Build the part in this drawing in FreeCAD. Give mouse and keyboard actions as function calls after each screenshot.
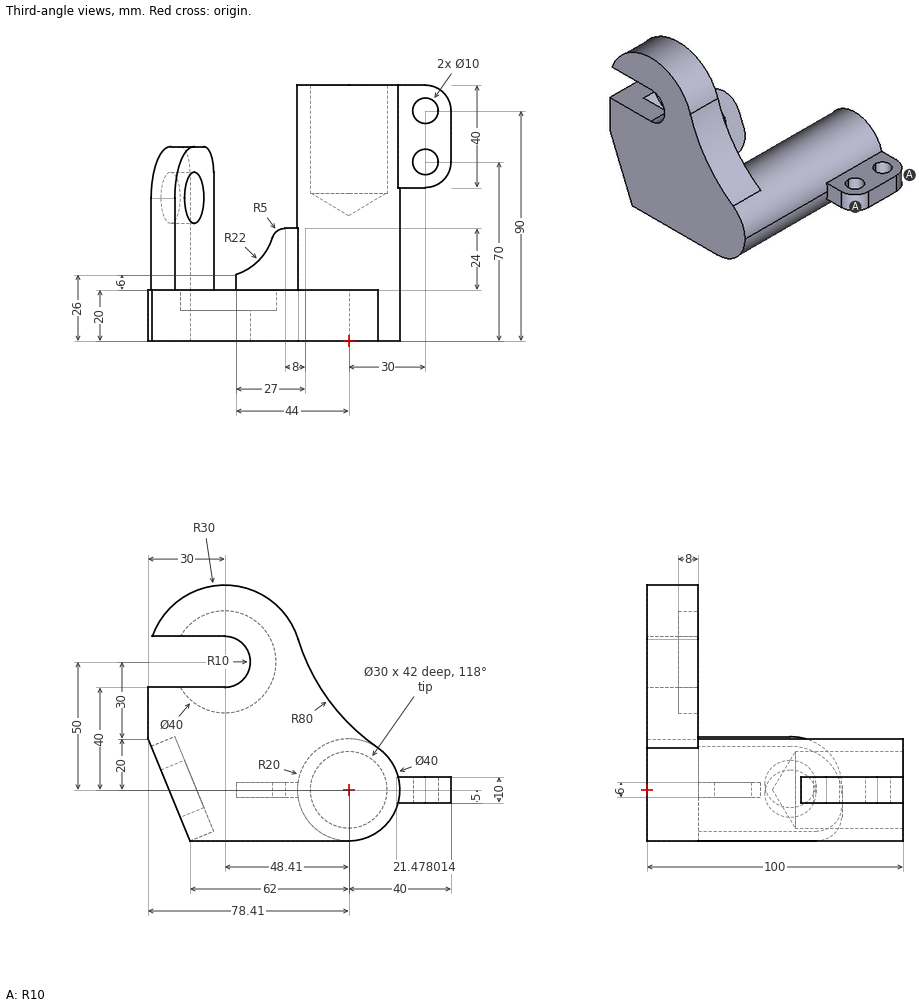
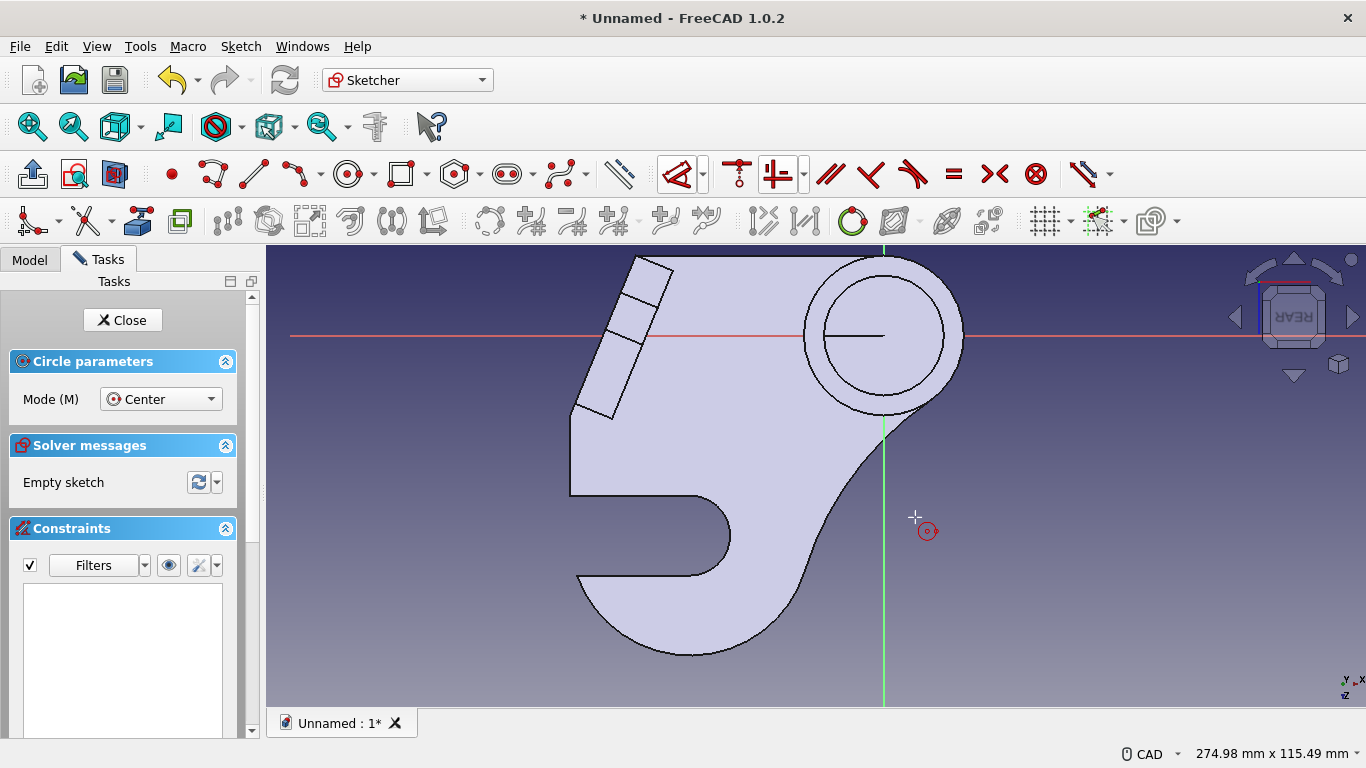
click(690, 536)
click(747, 479)
key(Escape)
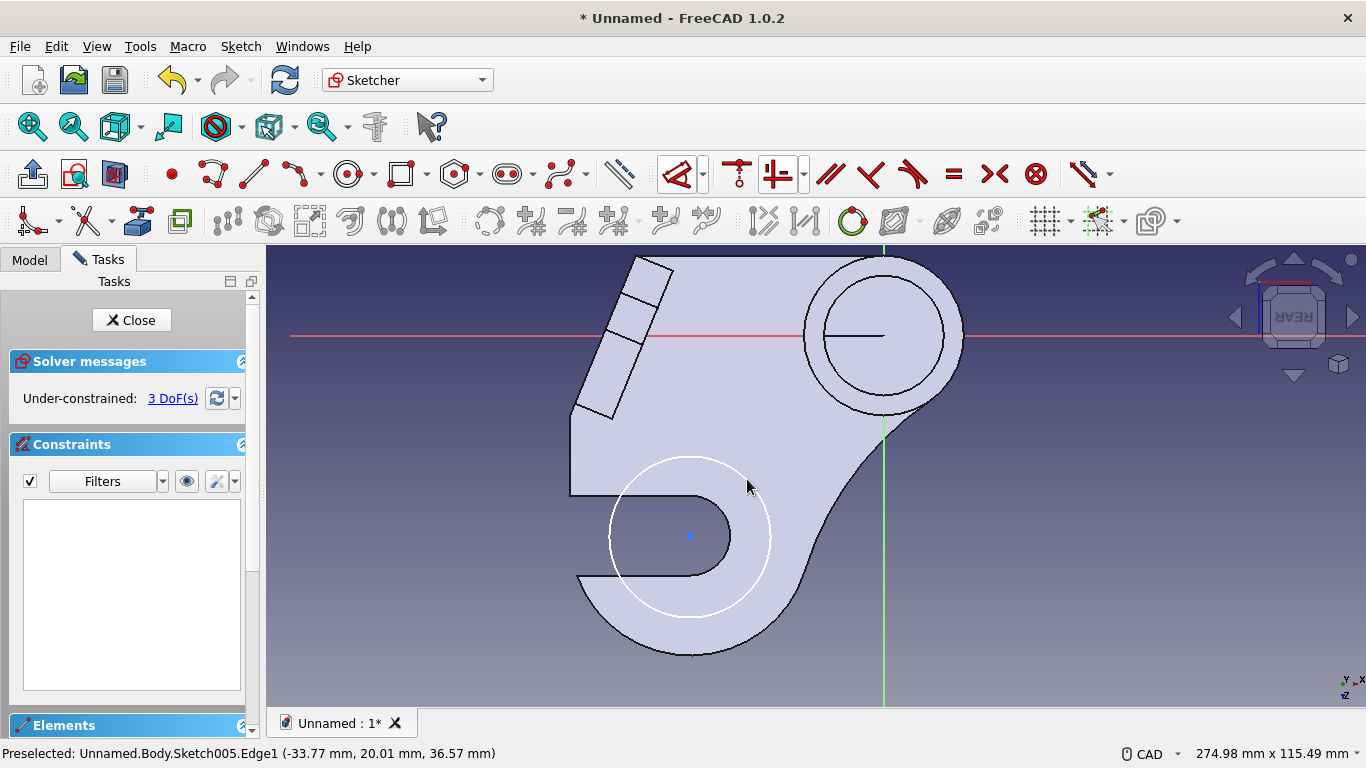
key(d)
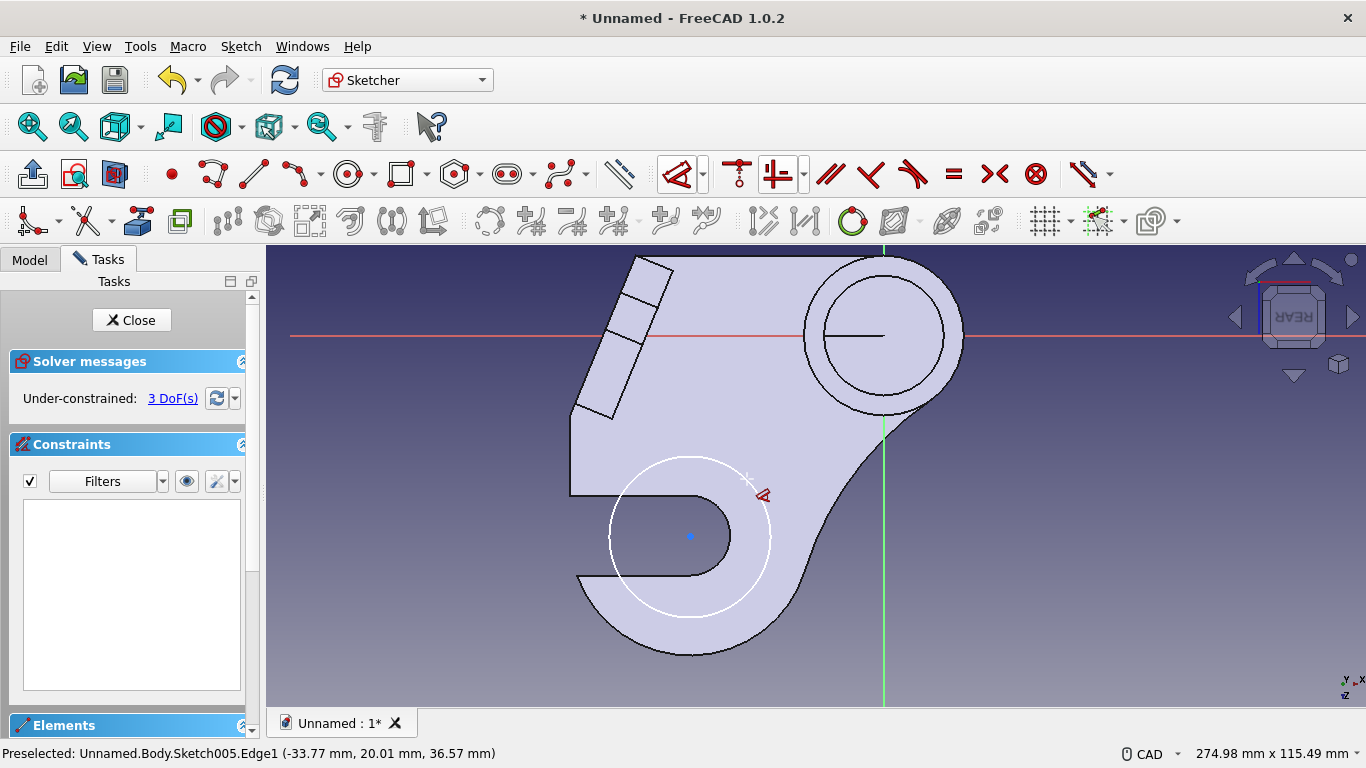
click(747, 480)
click(770, 457)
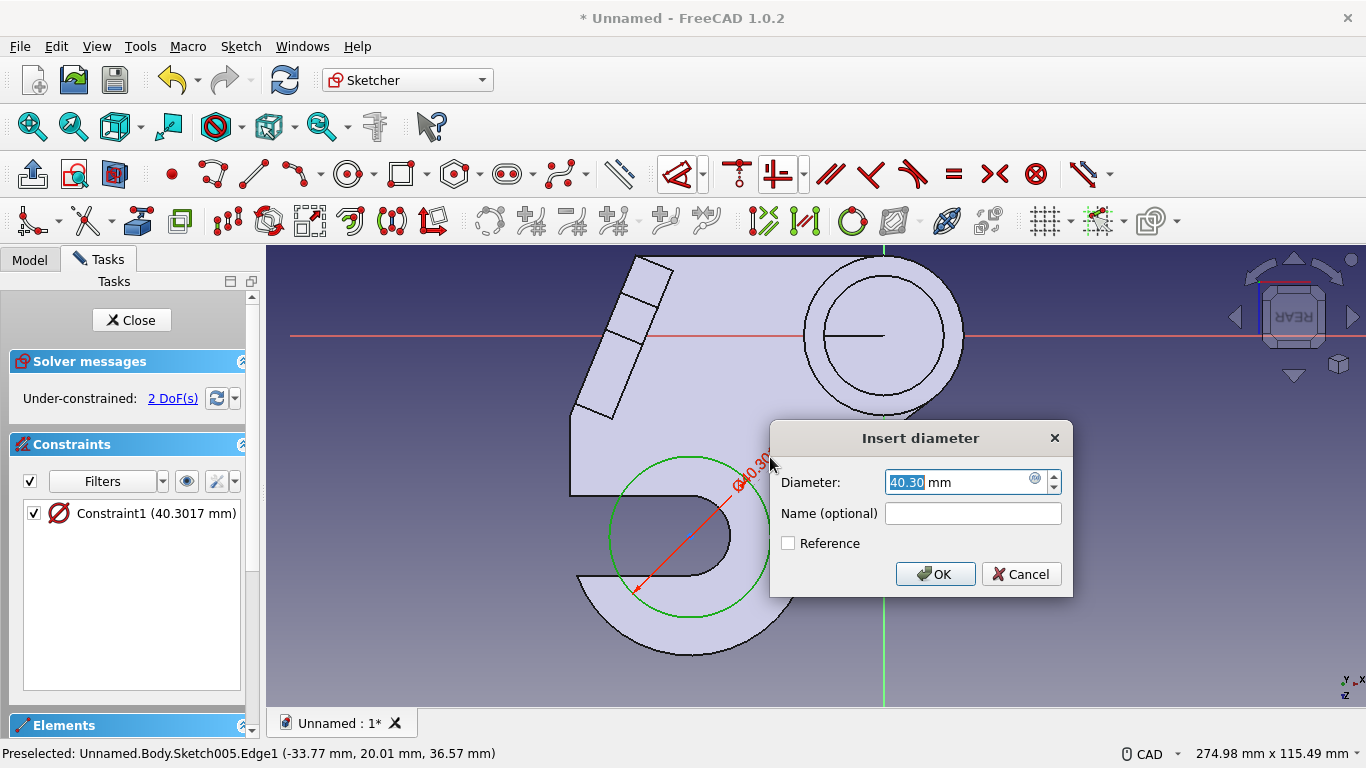
text(40)
key(Return)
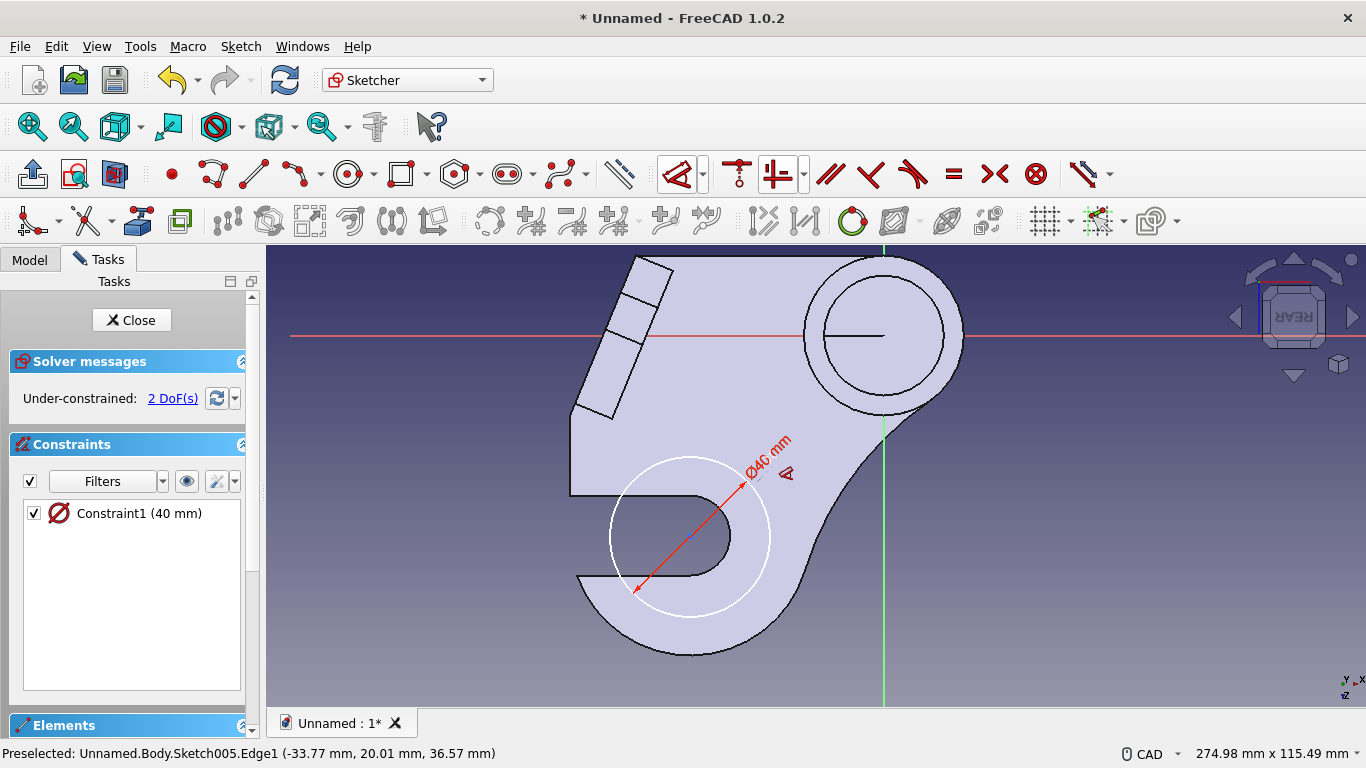
click(690, 537)
click(918, 436)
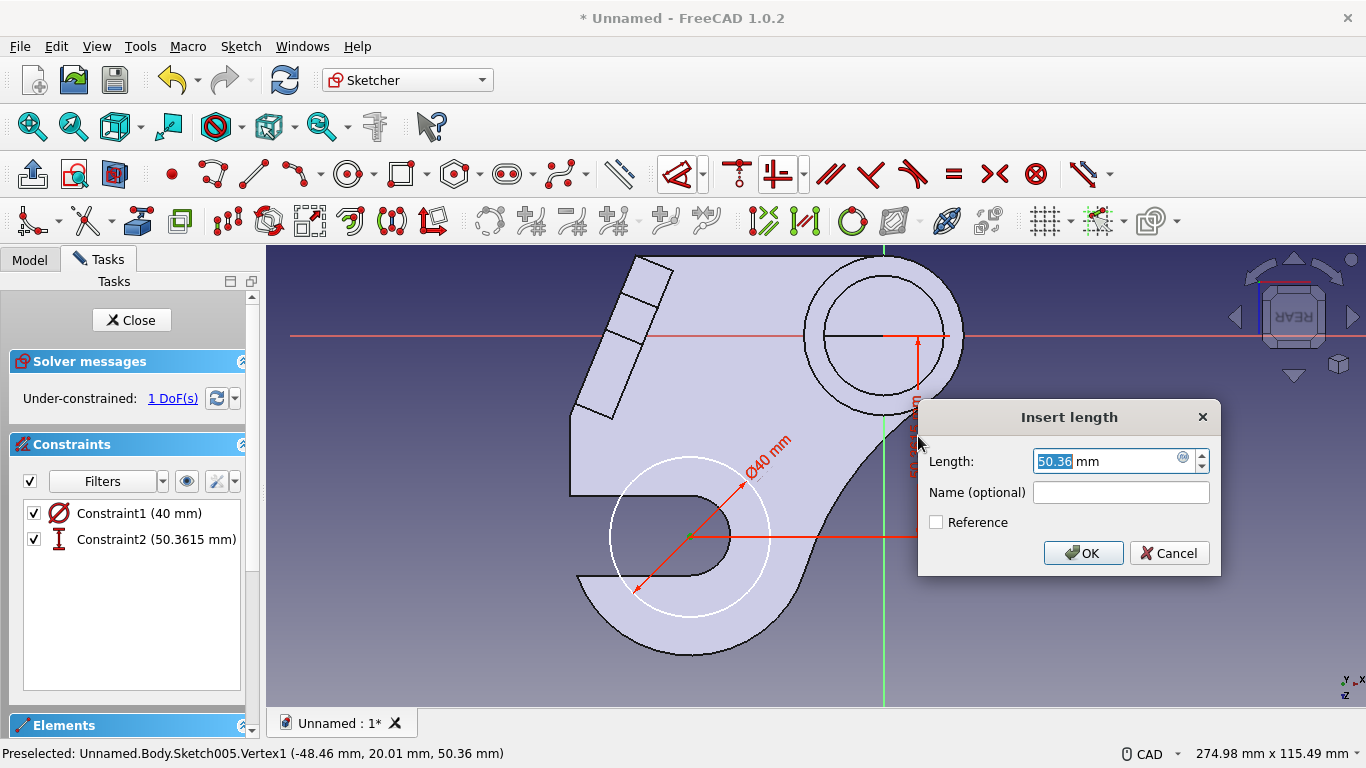
text(50)
key(Return)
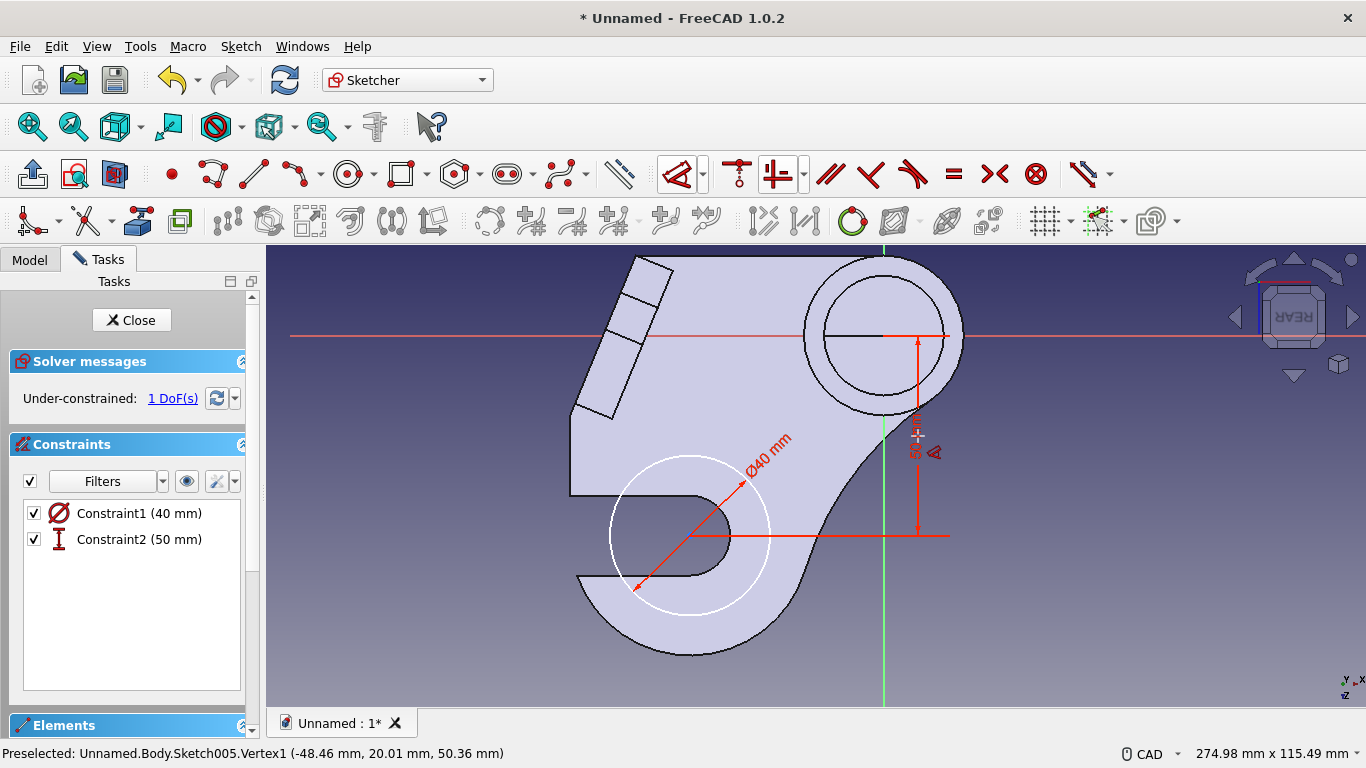
click(690, 536)
click(787, 302)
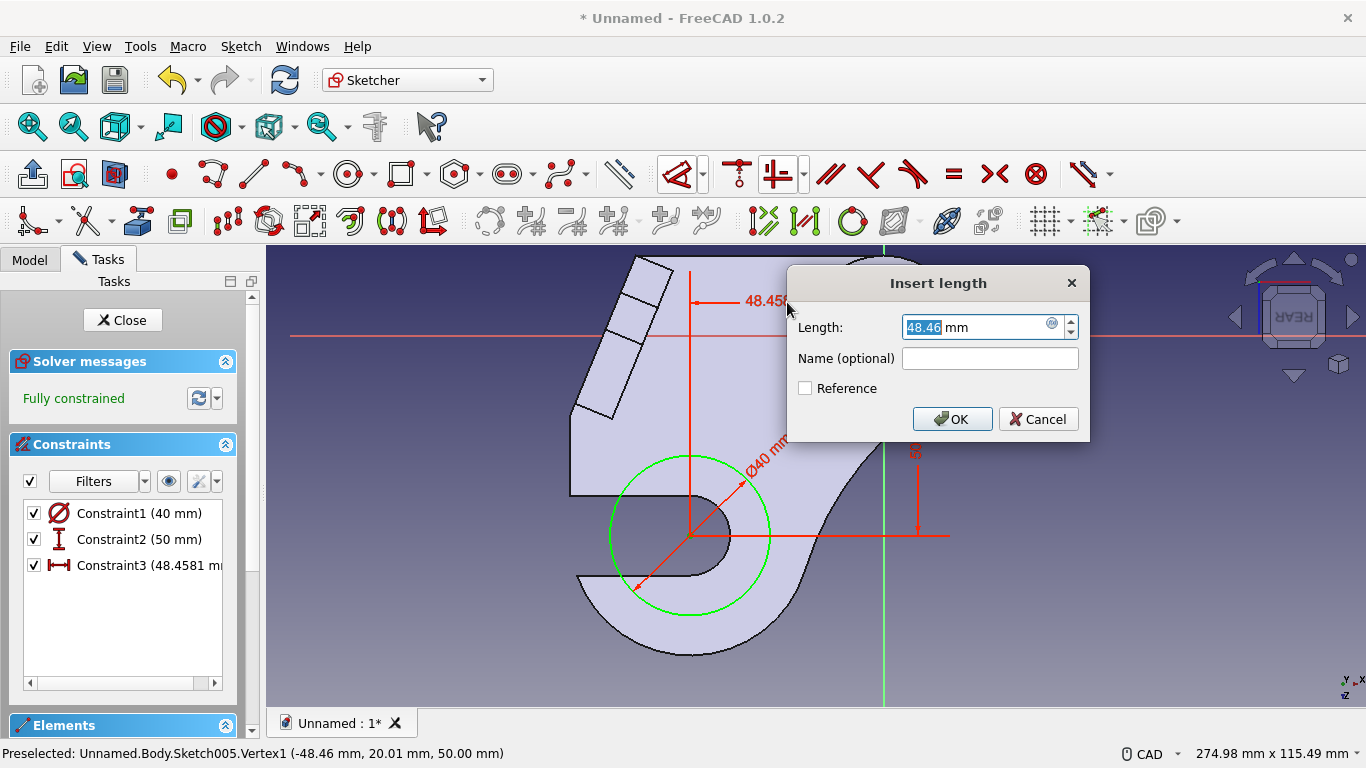
text(48.41)
key(Return)
key(Escape)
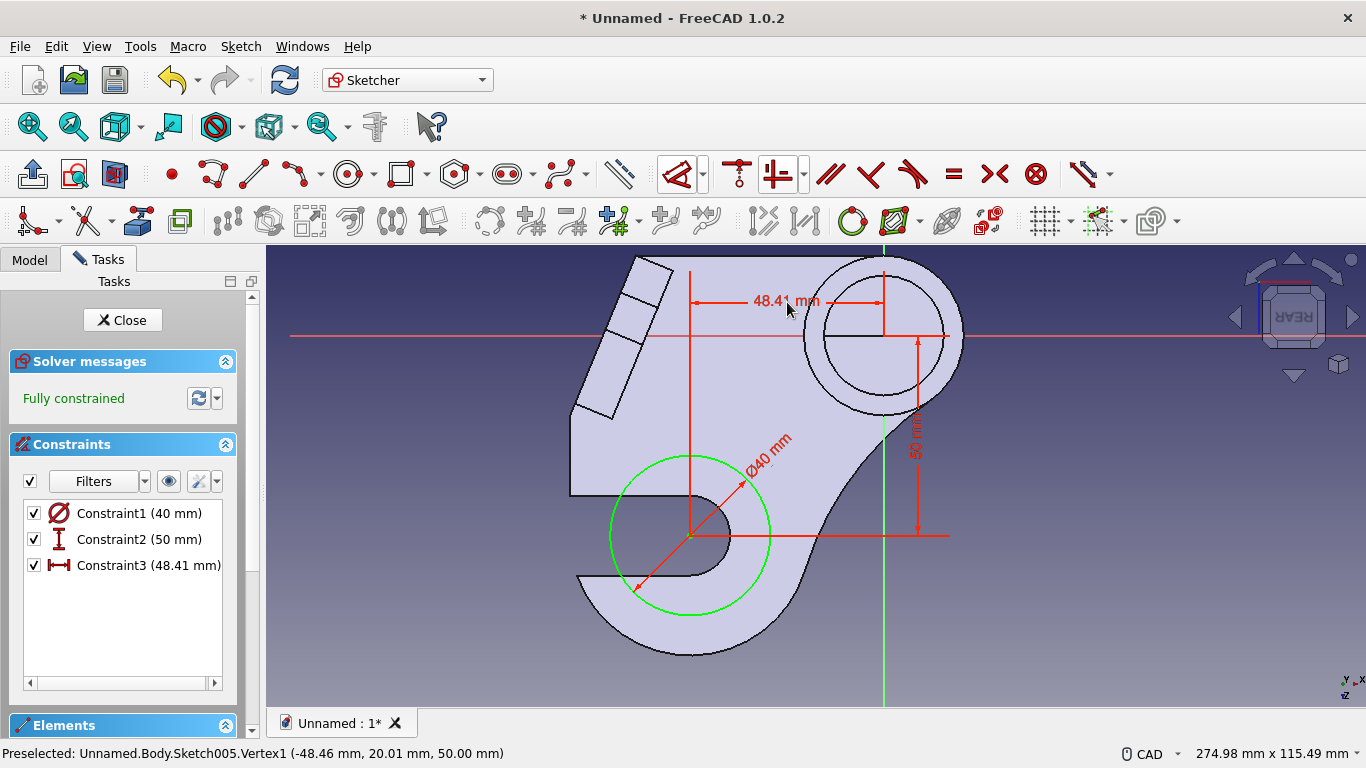
click(123, 320)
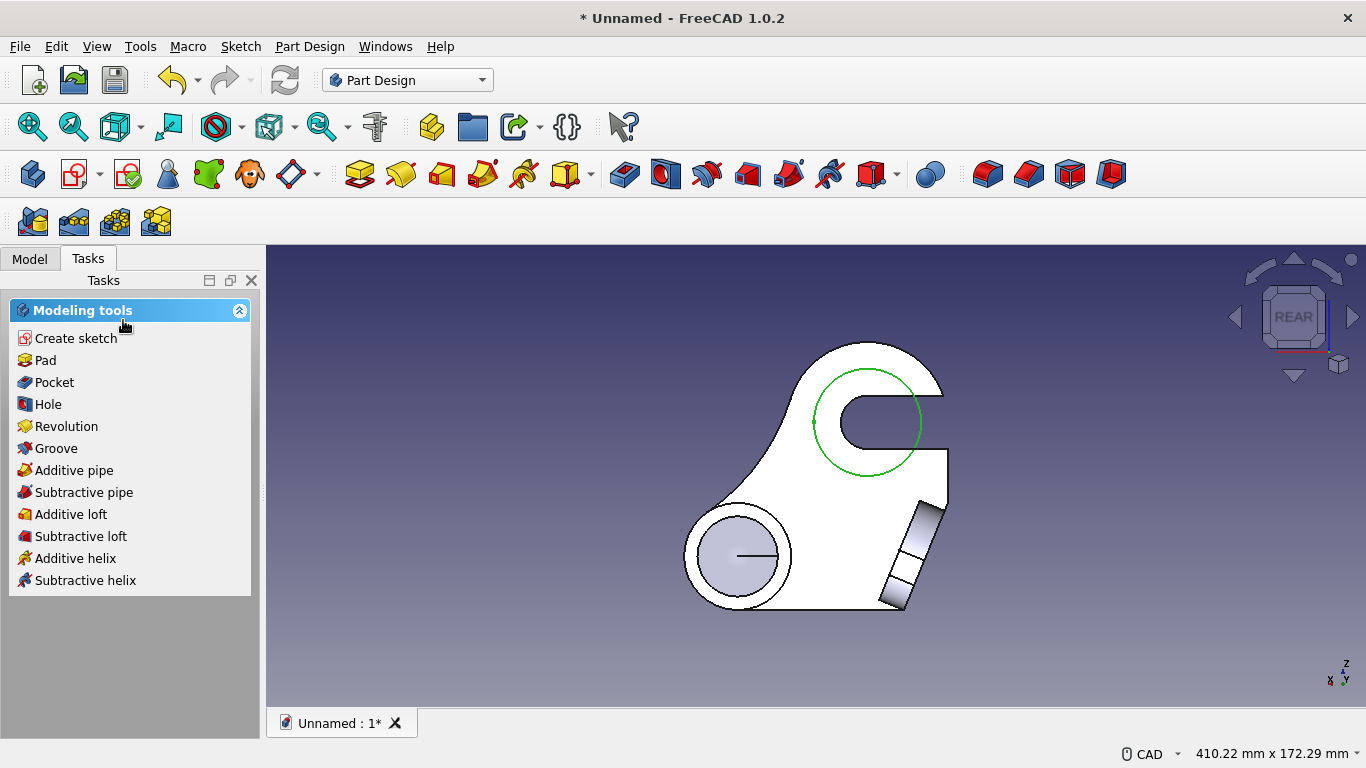
click(625, 174)